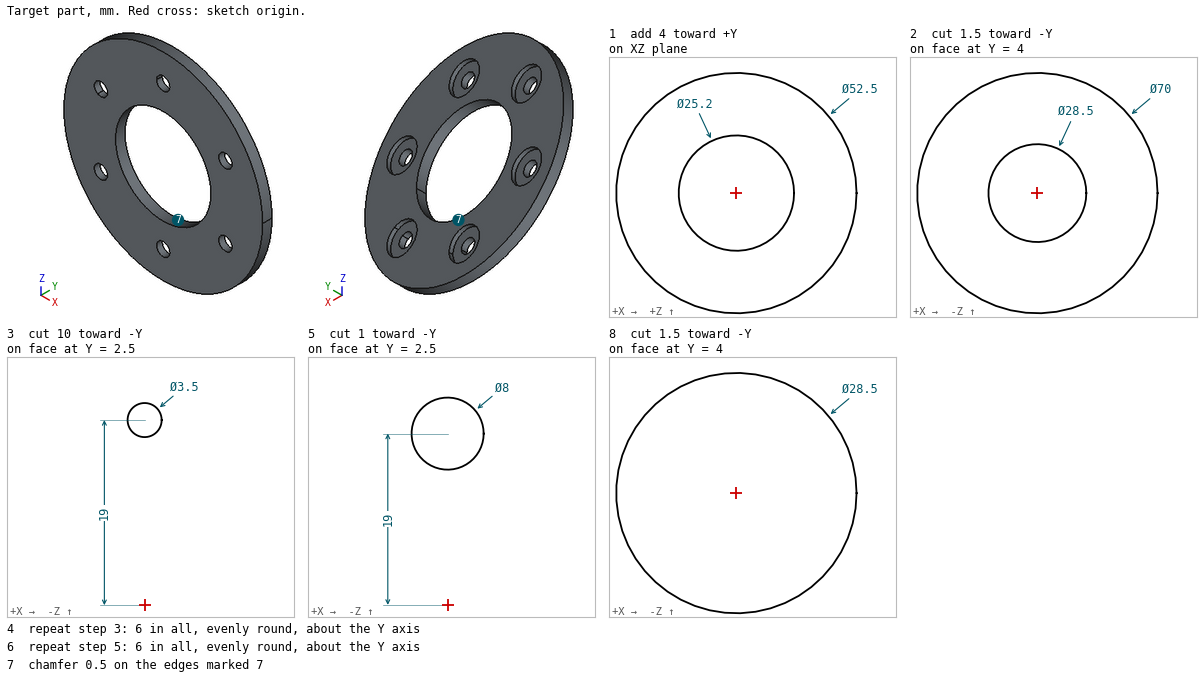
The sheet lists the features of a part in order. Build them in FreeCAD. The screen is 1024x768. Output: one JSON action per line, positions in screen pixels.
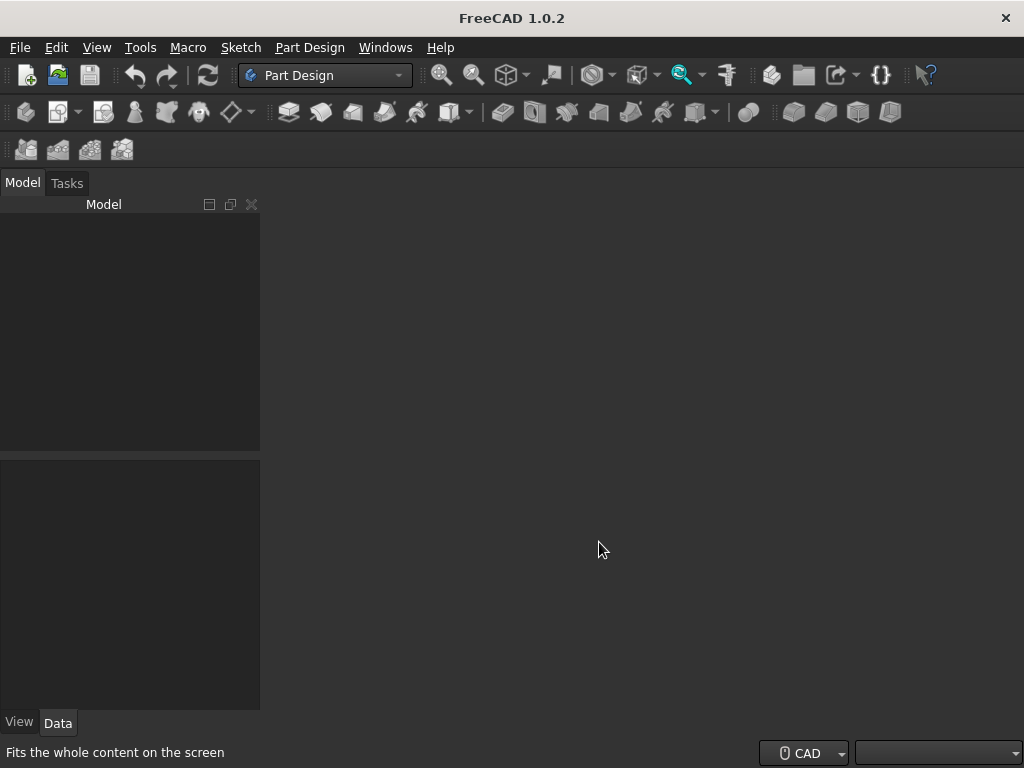
{"action": "left_click", "coordinate": [26, 76]}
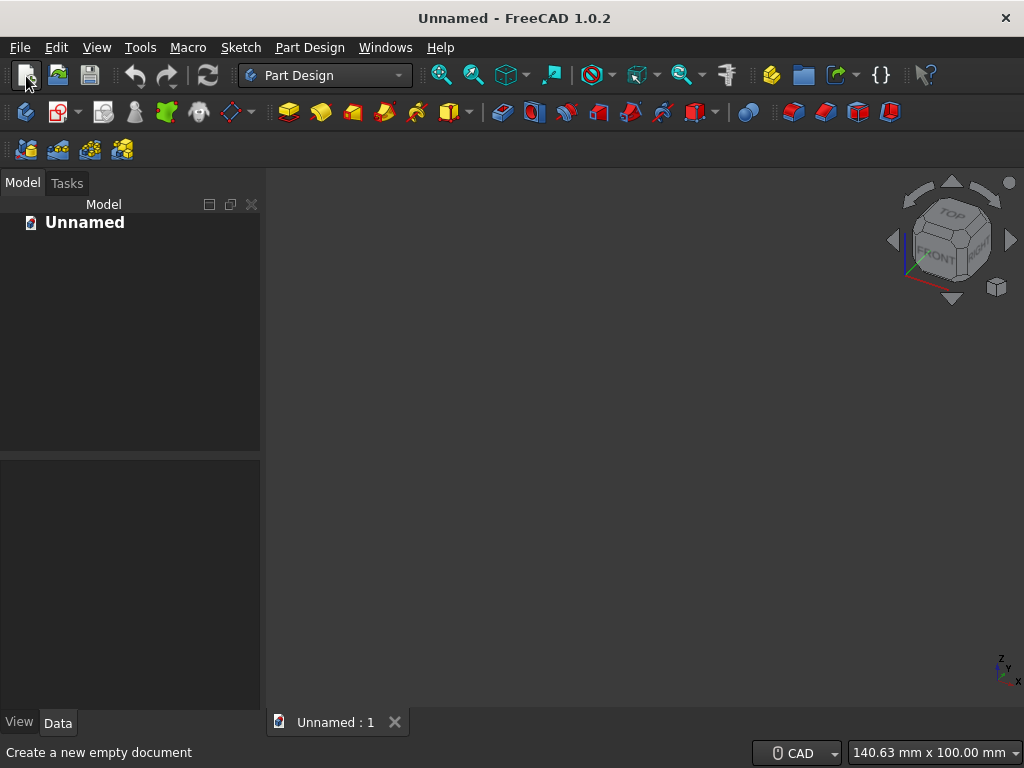
{"action": "left_click", "coordinate": [58, 112]}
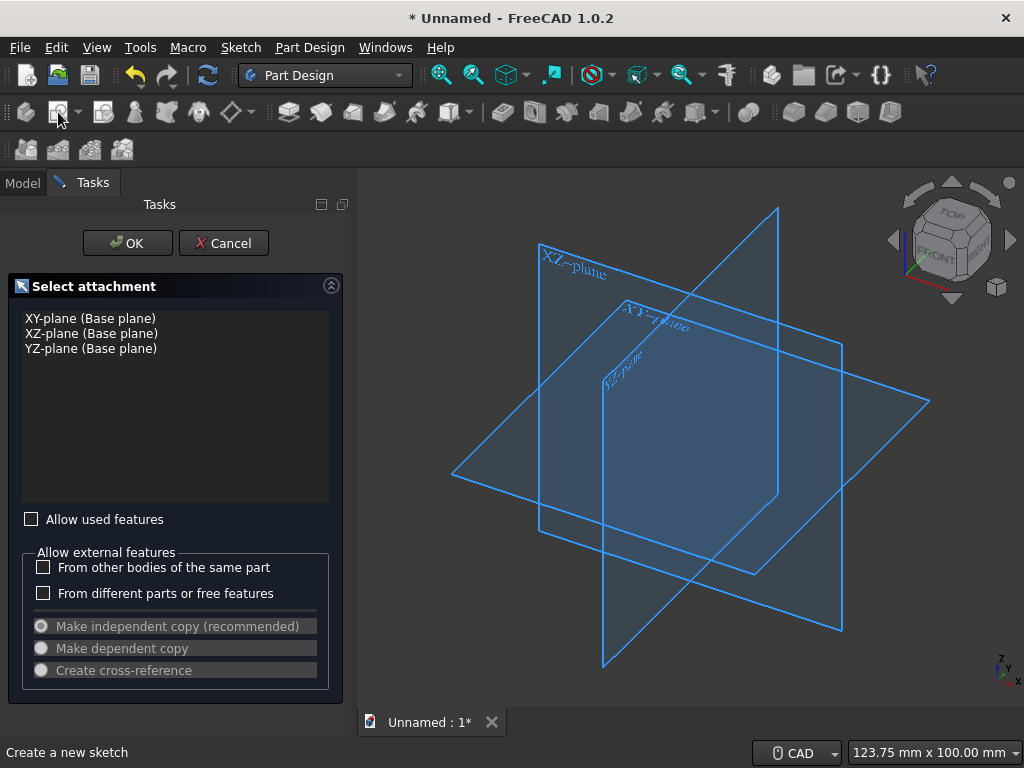
{"action": "left_click", "coordinate": [82, 334]}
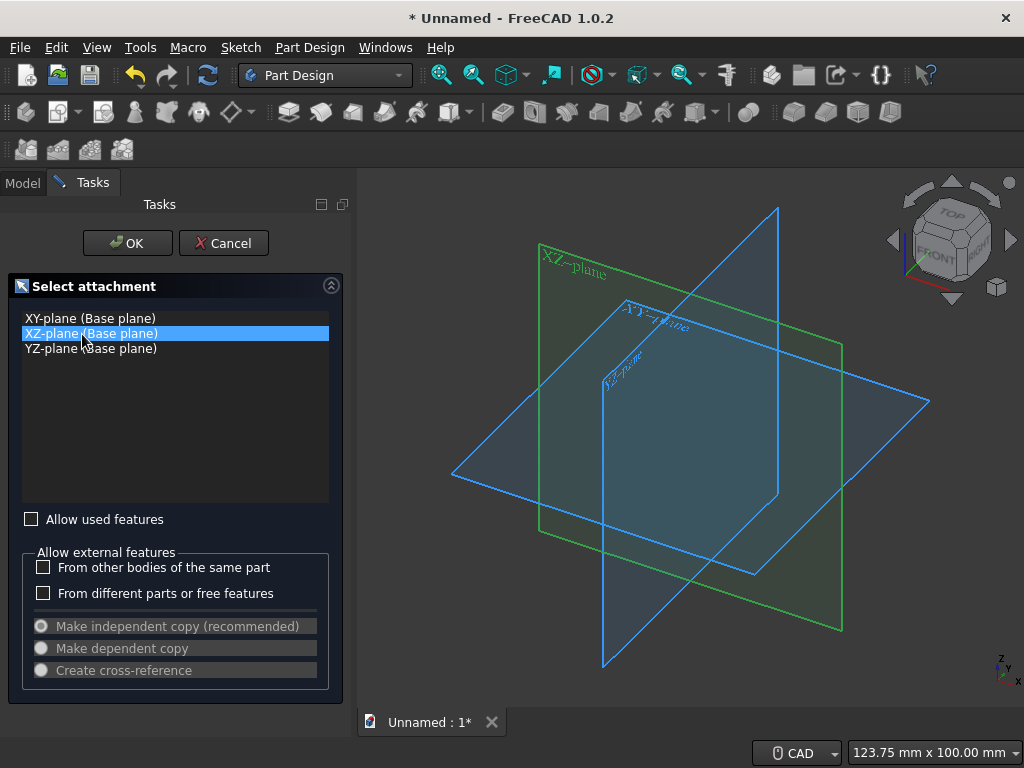
{"action": "left_click", "coordinate": [128, 243]}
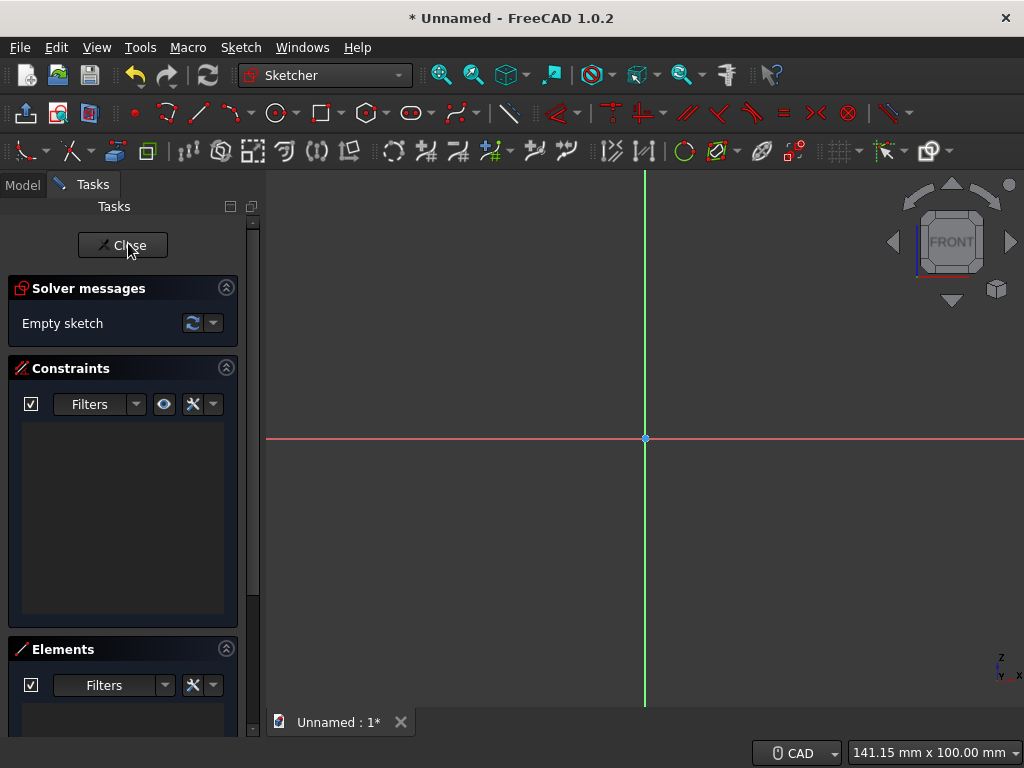
{"action": "left_click", "coordinate": [276, 114]}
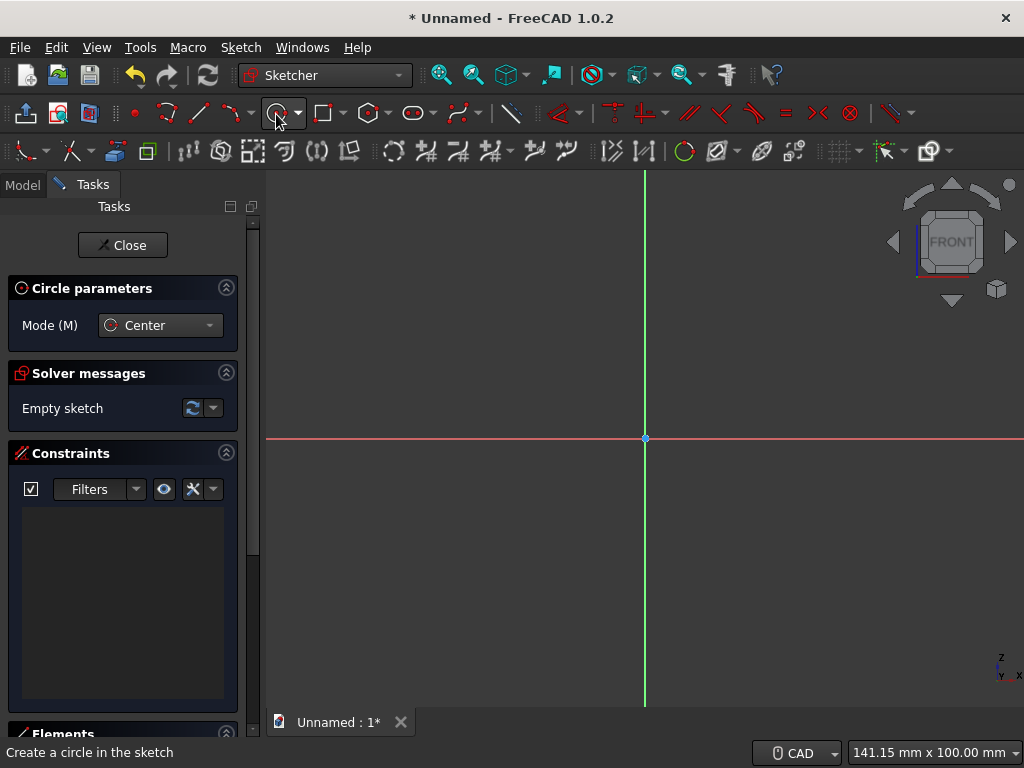
{"action": "left_click", "coordinate": [645, 438]}
{"action": "mouse_move", "coordinate": [745, 339]}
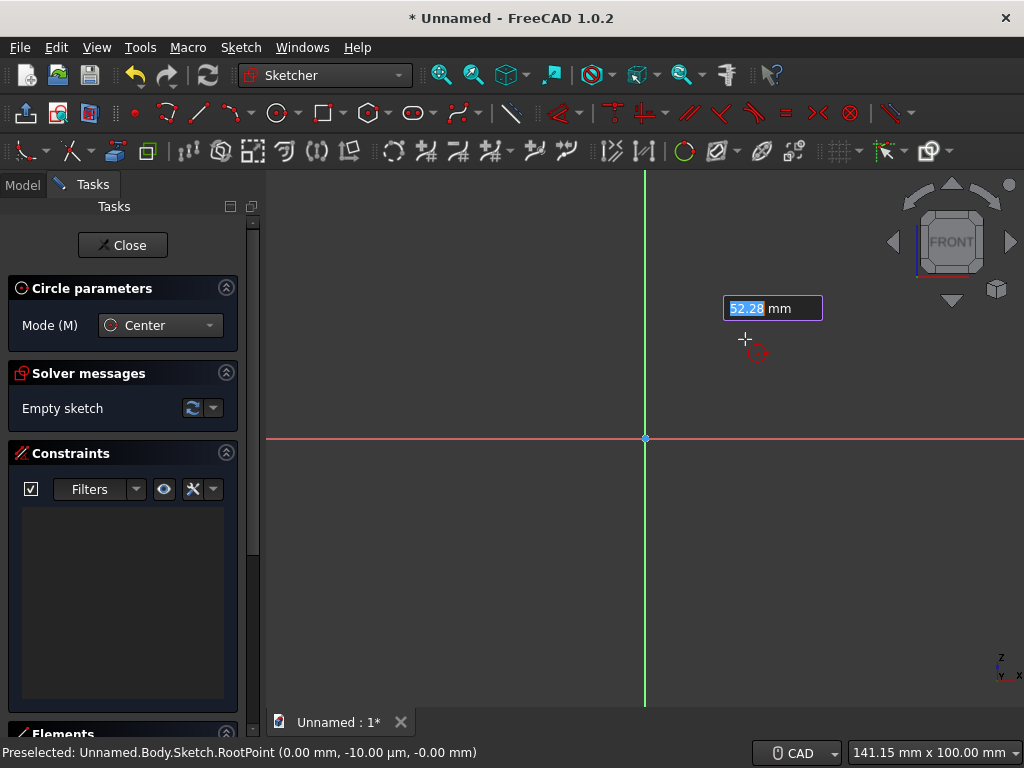
{"action": "type", "text": "52.5"}
{"action": "key", "text": "Return"}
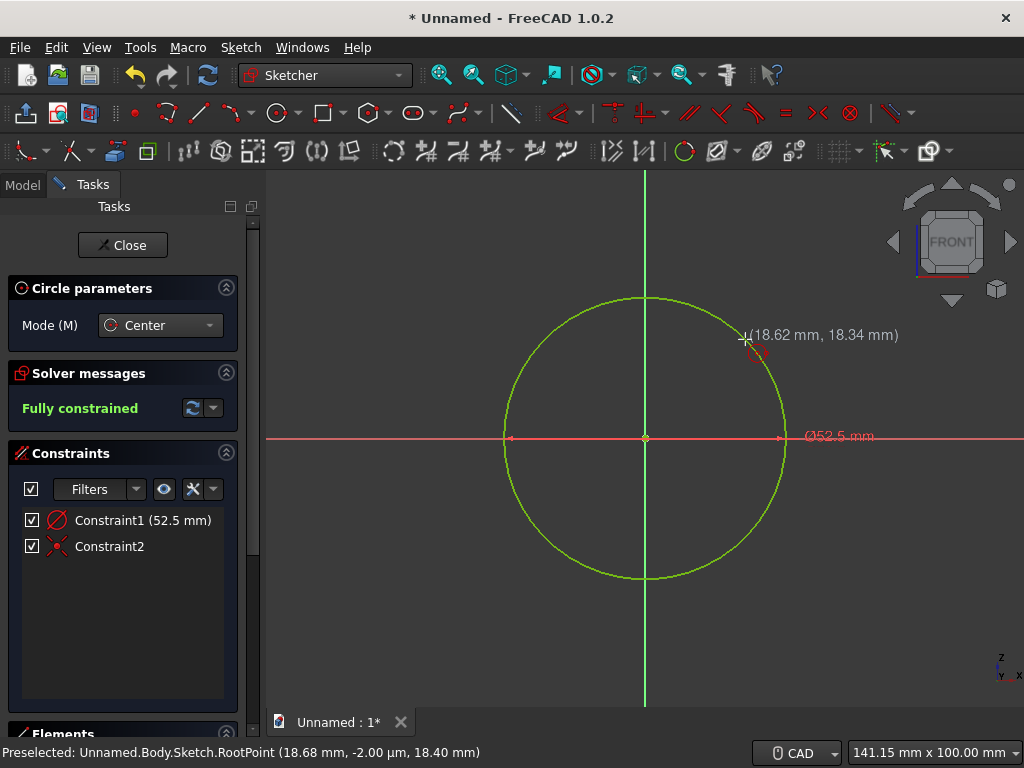
{"action": "left_click", "coordinate": [645, 438]}
{"action": "mouse_move", "coordinate": [693, 391]}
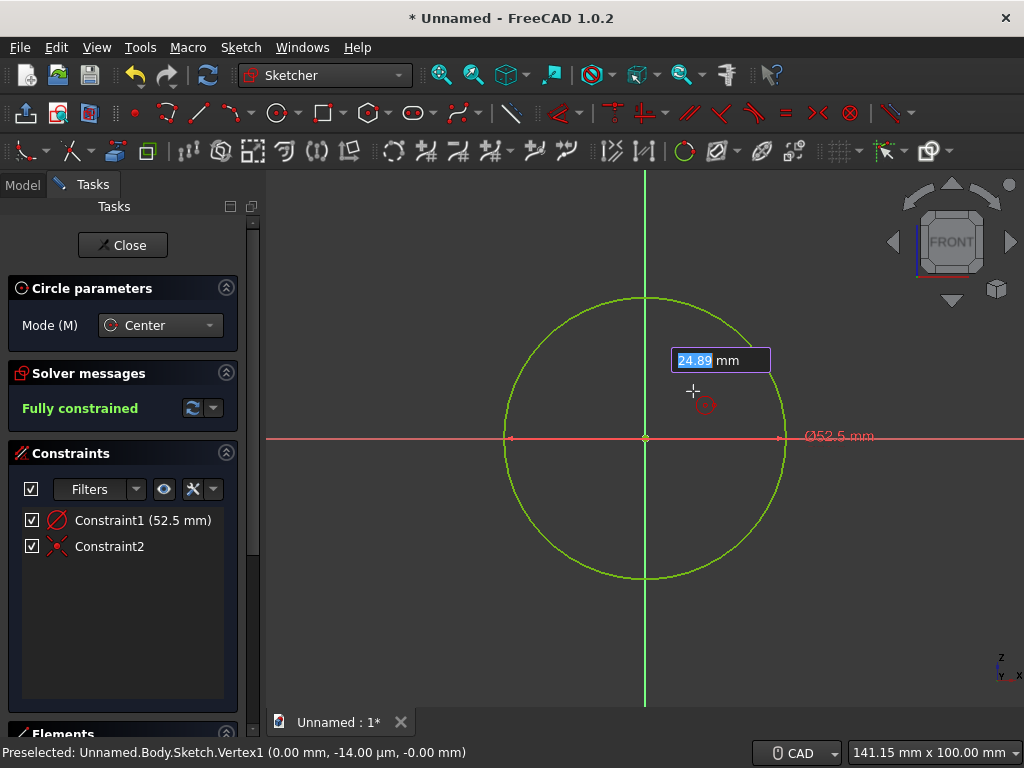
{"action": "type", "text": "25.2"}
{"action": "key", "text": "Return"}
{"action": "key", "text": "Escape"}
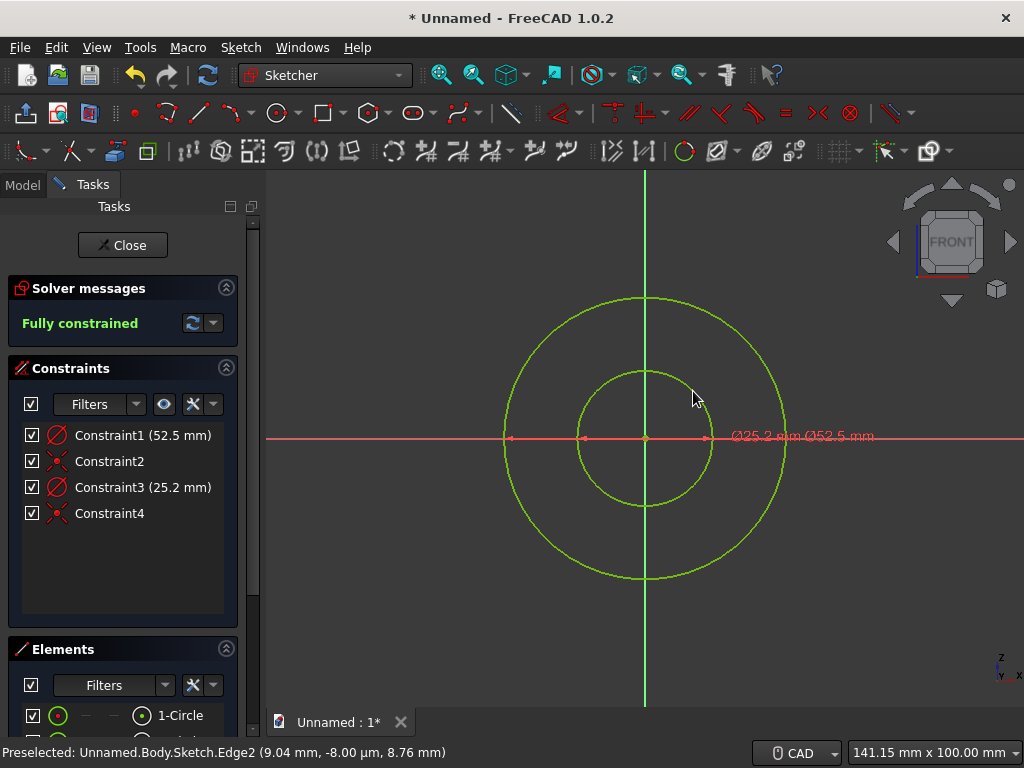
{"action": "left_click", "coordinate": [123, 245]}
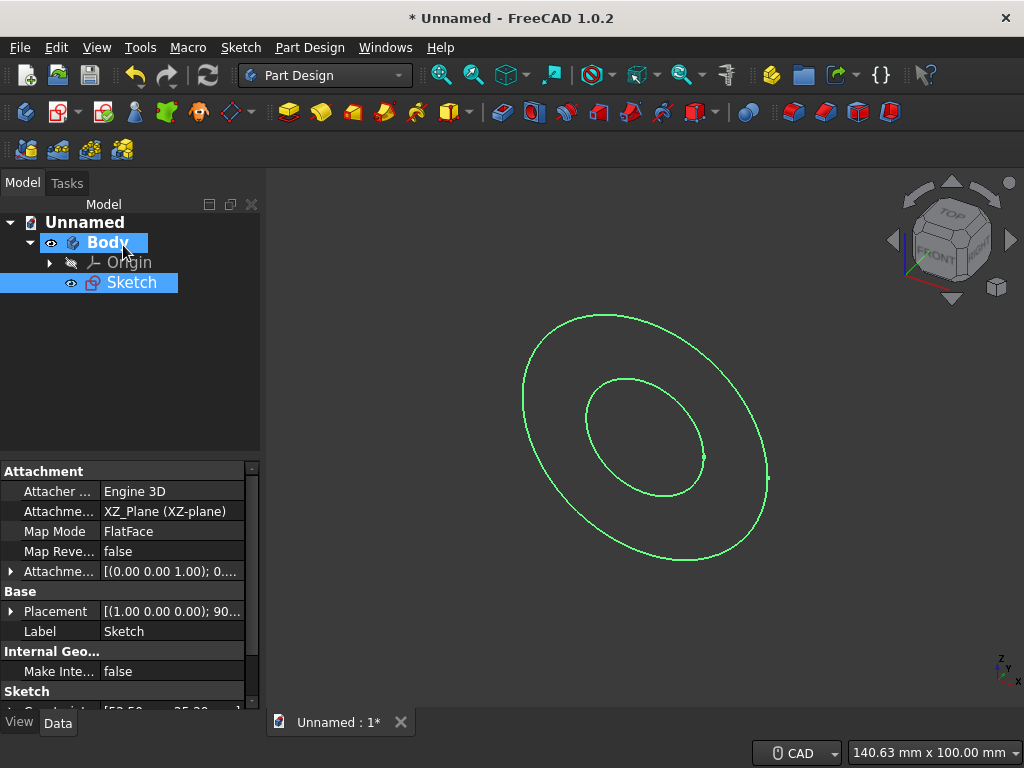
{"action": "left_click", "coordinate": [290, 112]}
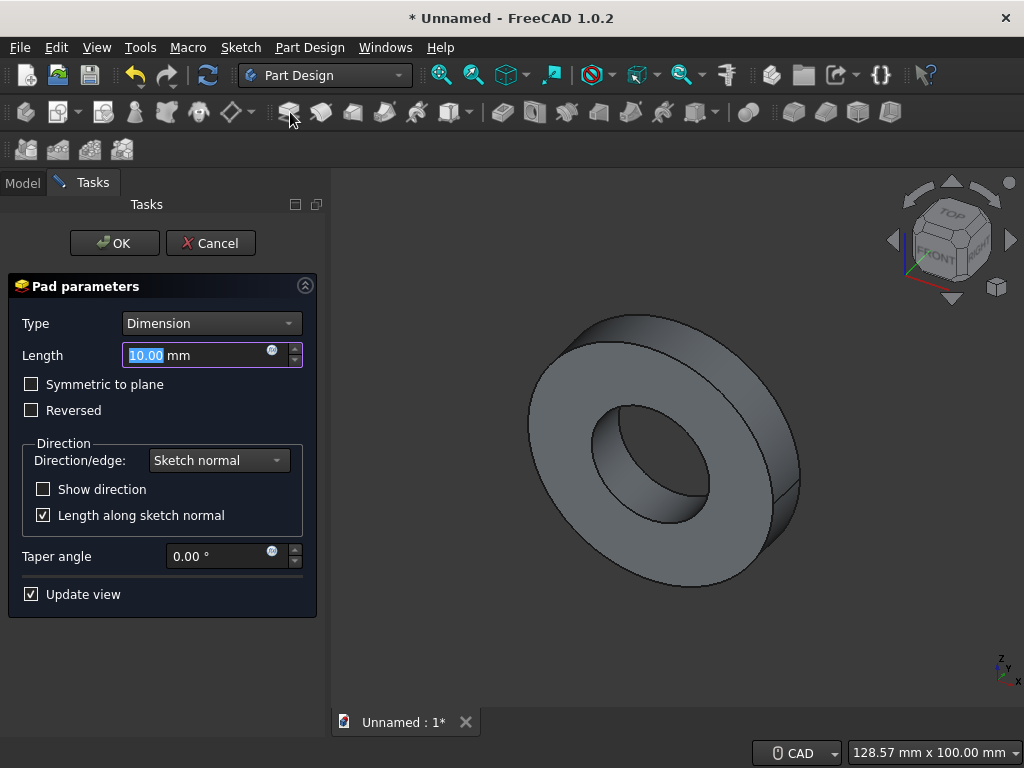
{"action": "type", "text": "4"}
{"action": "key", "text": "Tab"}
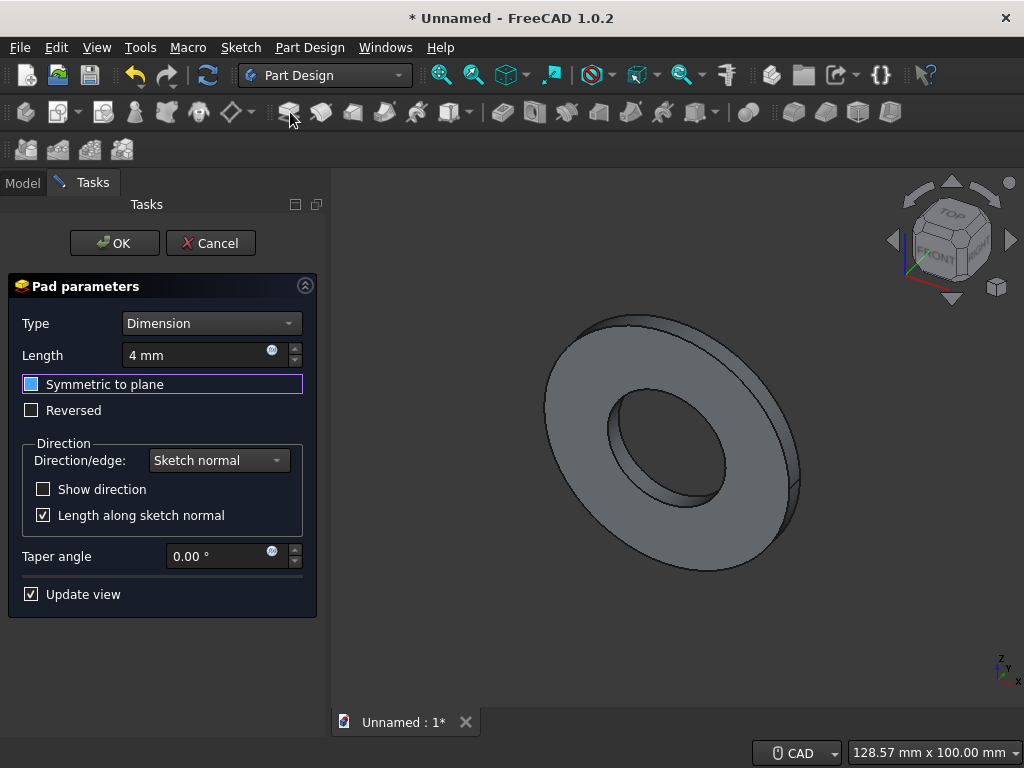
{"action": "left_click", "coordinate": [30, 410]}